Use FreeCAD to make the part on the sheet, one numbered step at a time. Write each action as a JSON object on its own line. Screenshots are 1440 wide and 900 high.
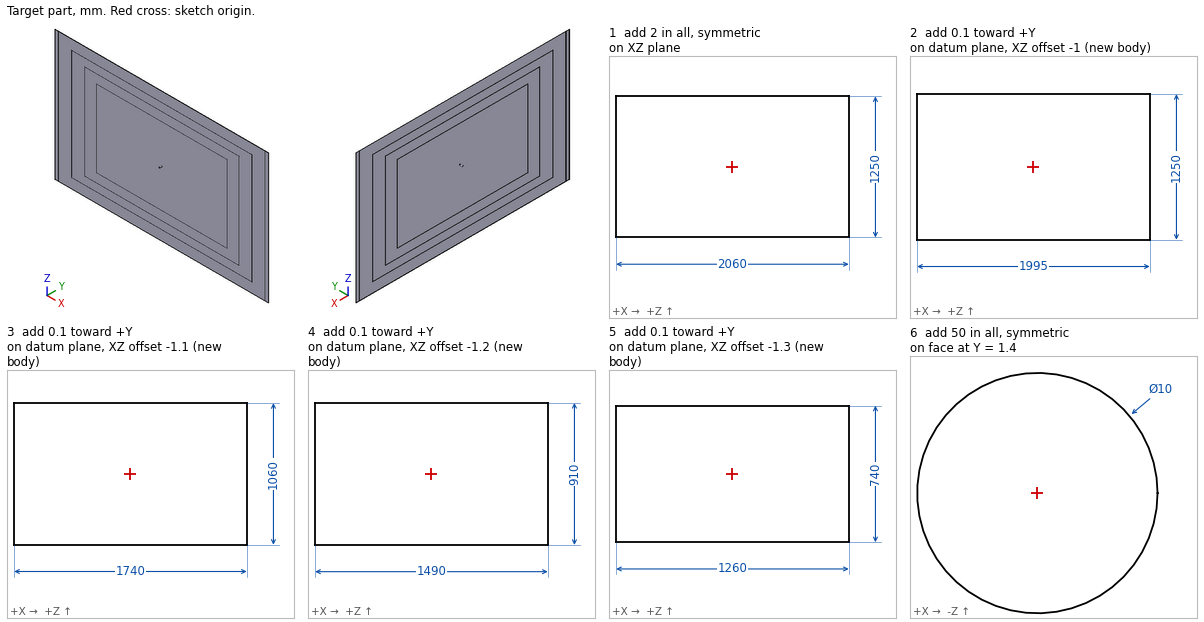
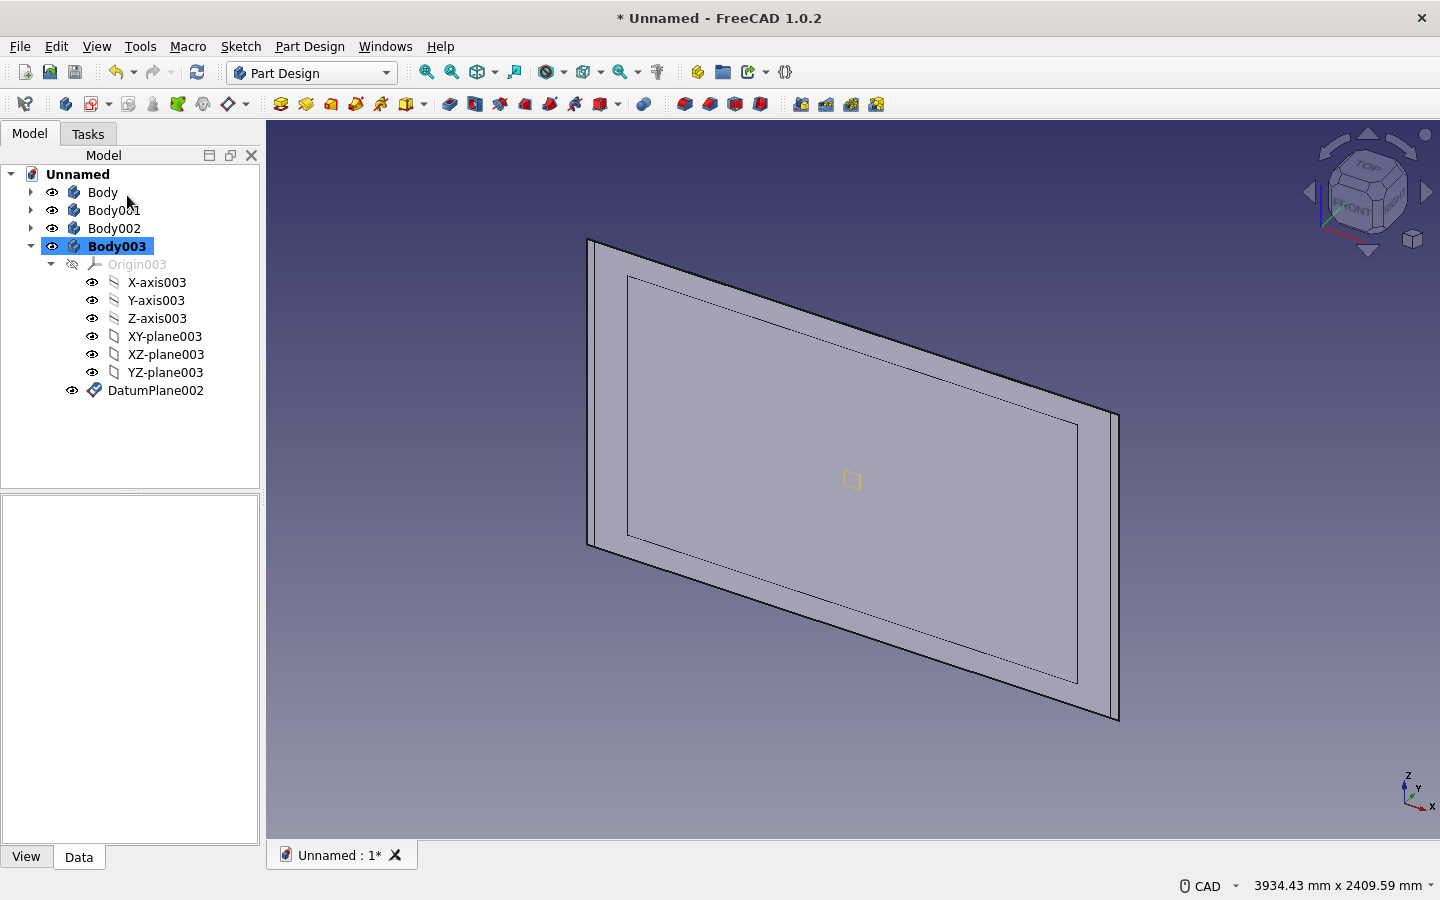
{"action": "left_click", "coordinate": [117, 390]}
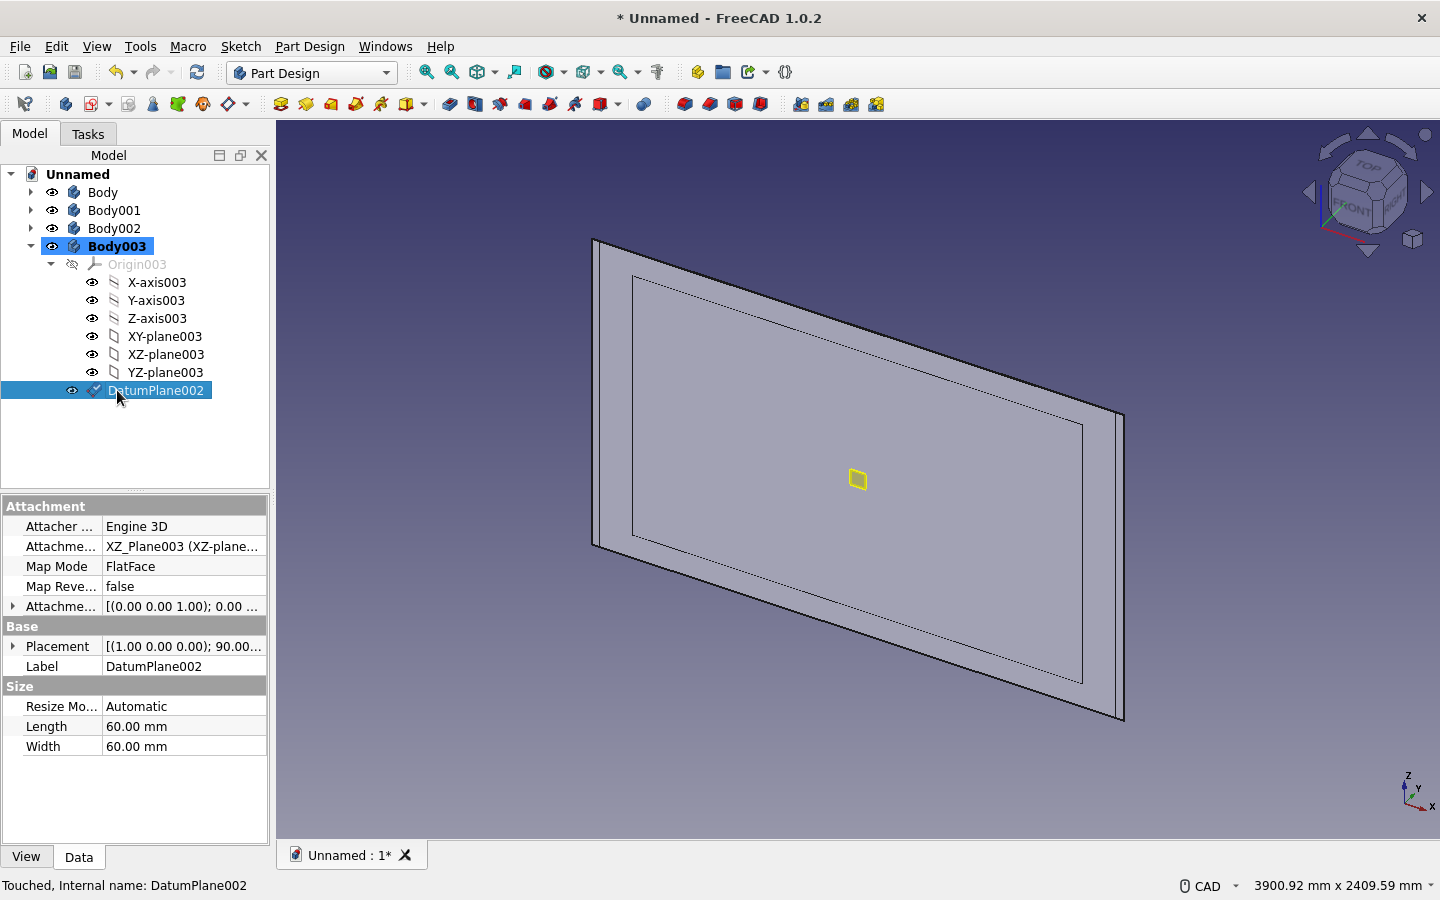
{"action": "left_click", "coordinate": [90, 104]}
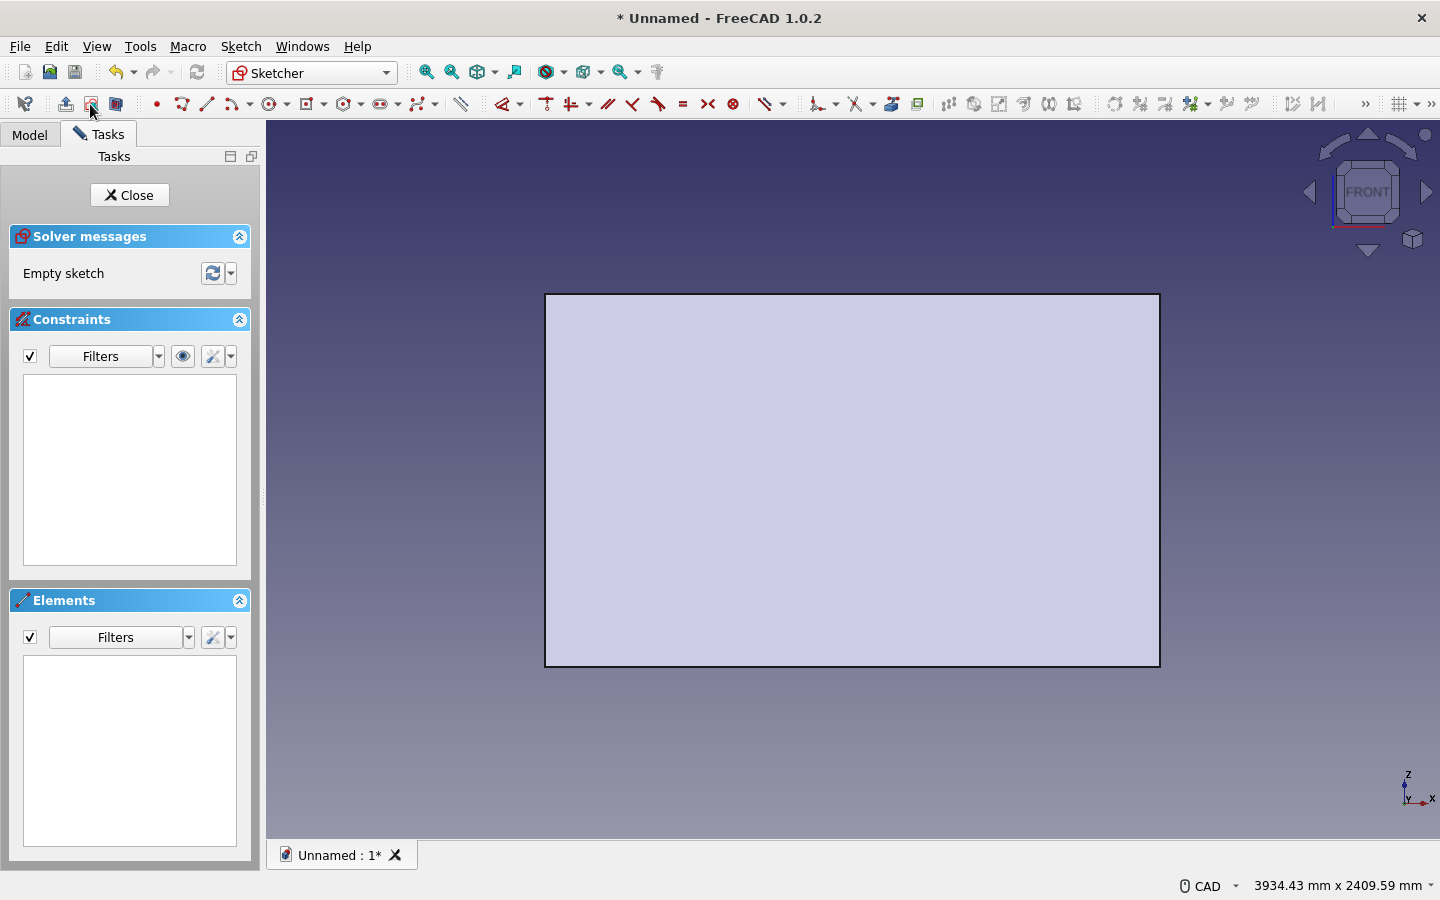
{"action": "scroll", "coordinate": [991, 481], "scroll_direction": "up", "scroll_amount": 2}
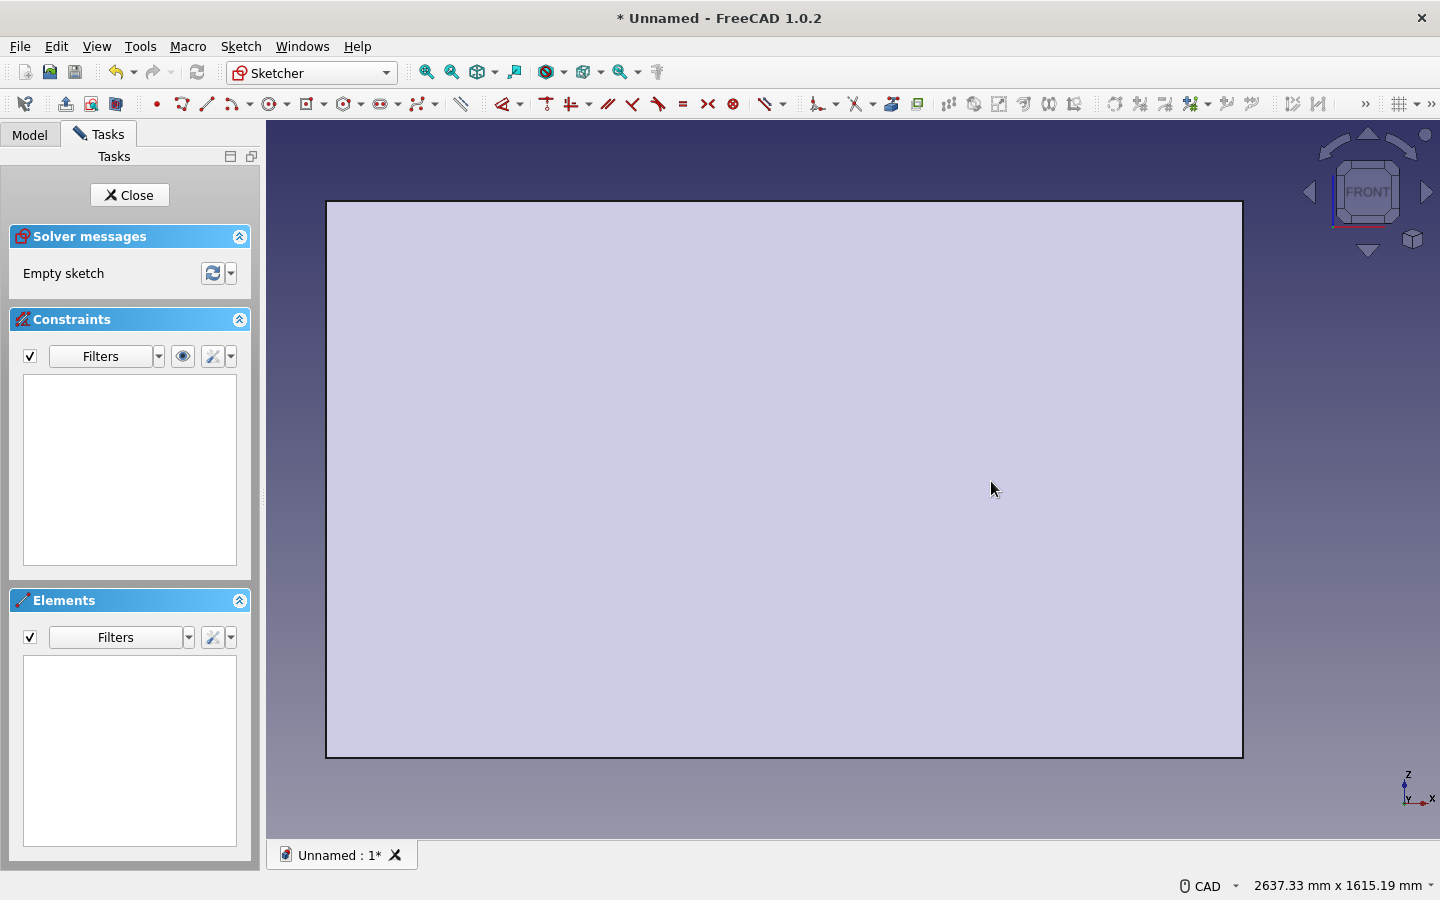
{"action": "left_click", "coordinate": [306, 104]}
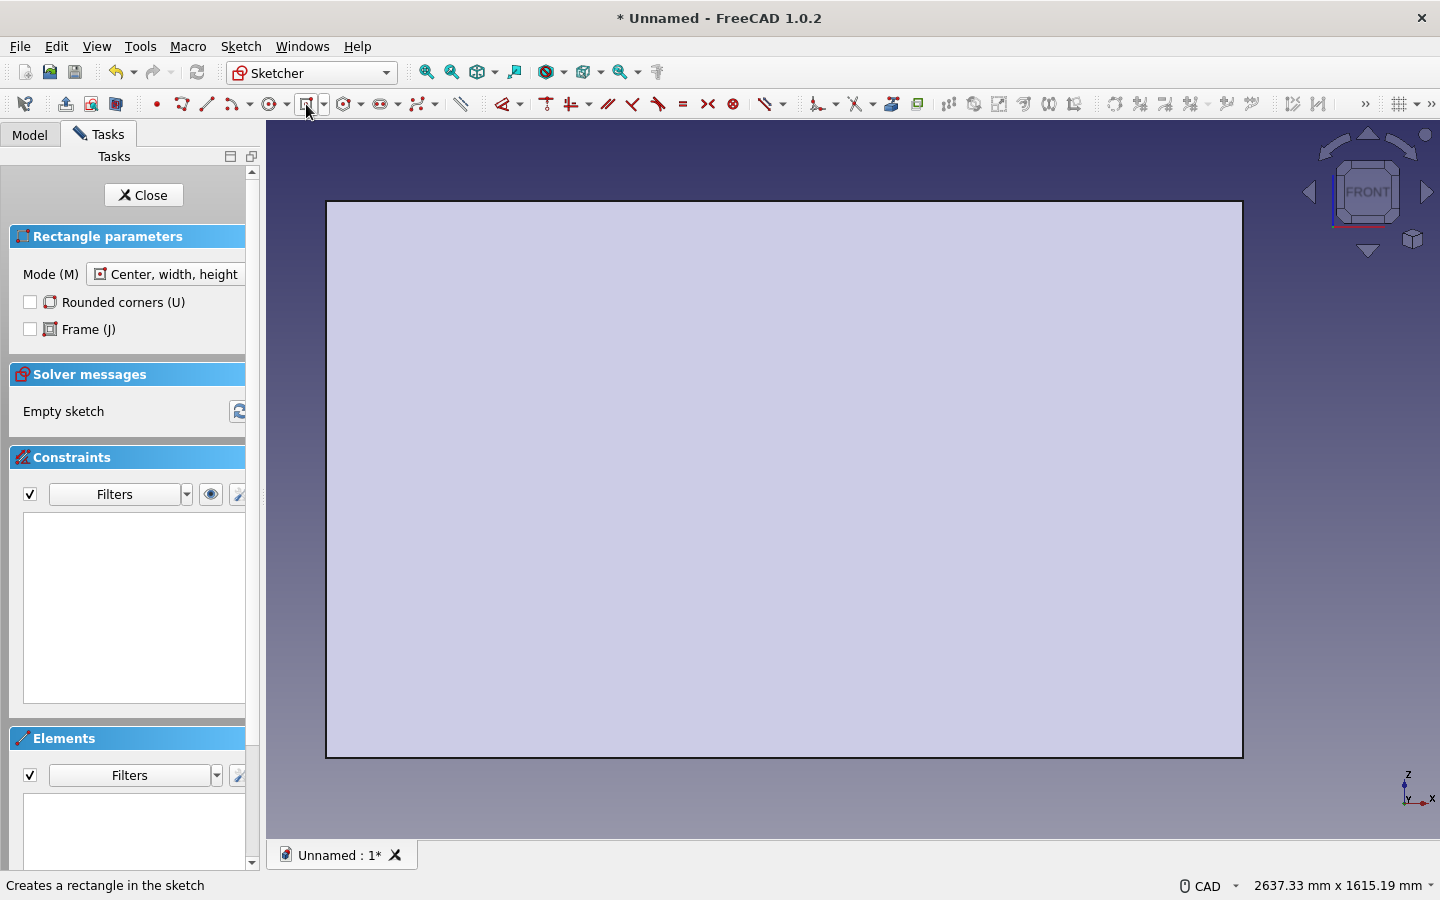
{"action": "left_click", "coordinate": [784, 479]}
{"action": "mouse_move", "coordinate": [1116, 277]}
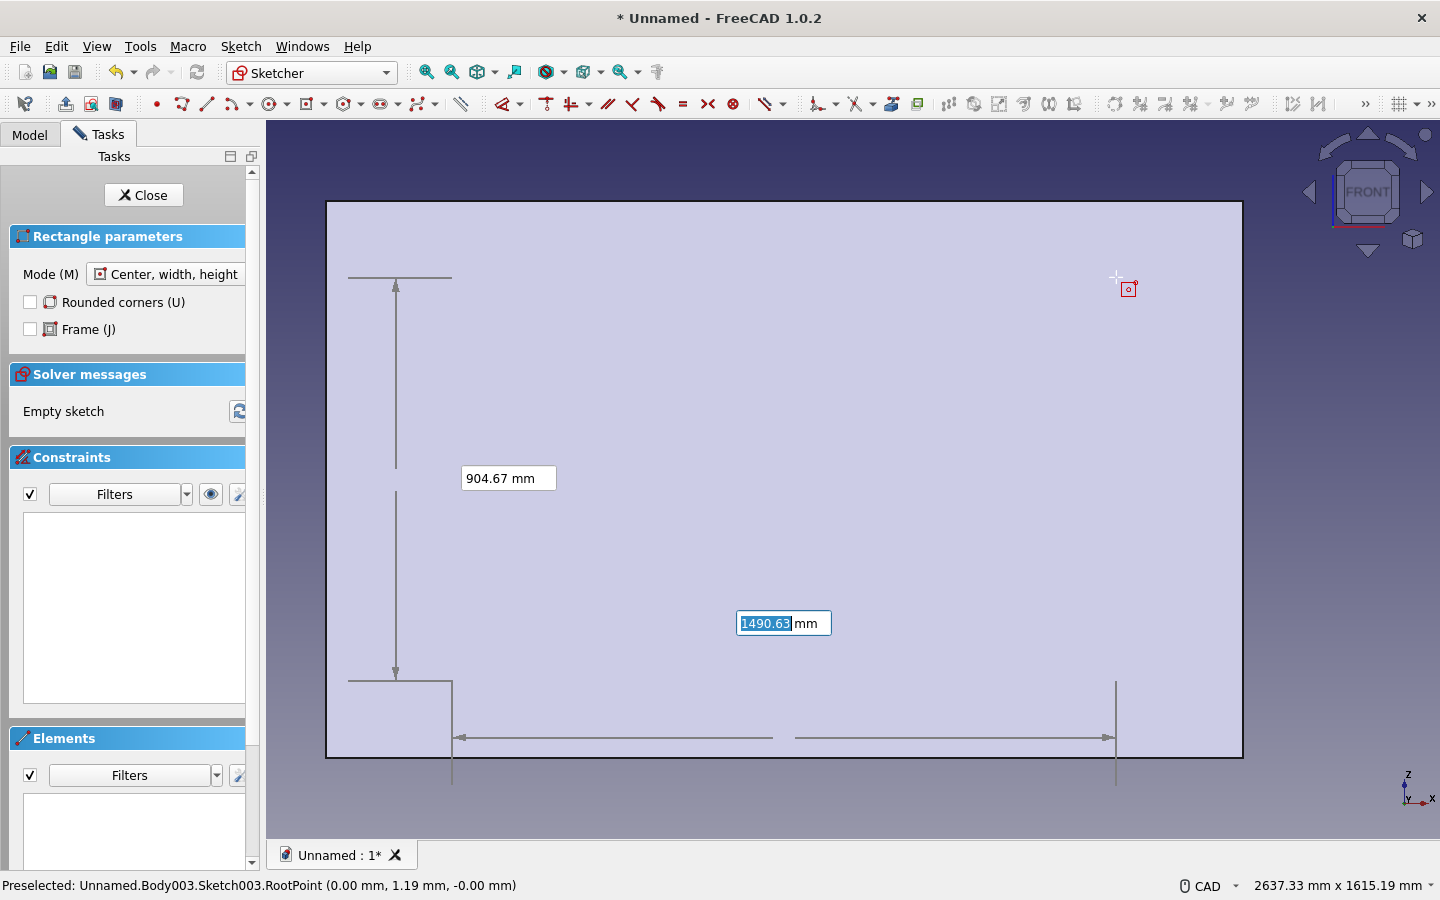
{"action": "type", "text": "1490"}
{"action": "key", "text": "Tab"}
{"action": "type", "text": "910"}
{"action": "key", "text": "Return"}
{"action": "key", "text": "Escape"}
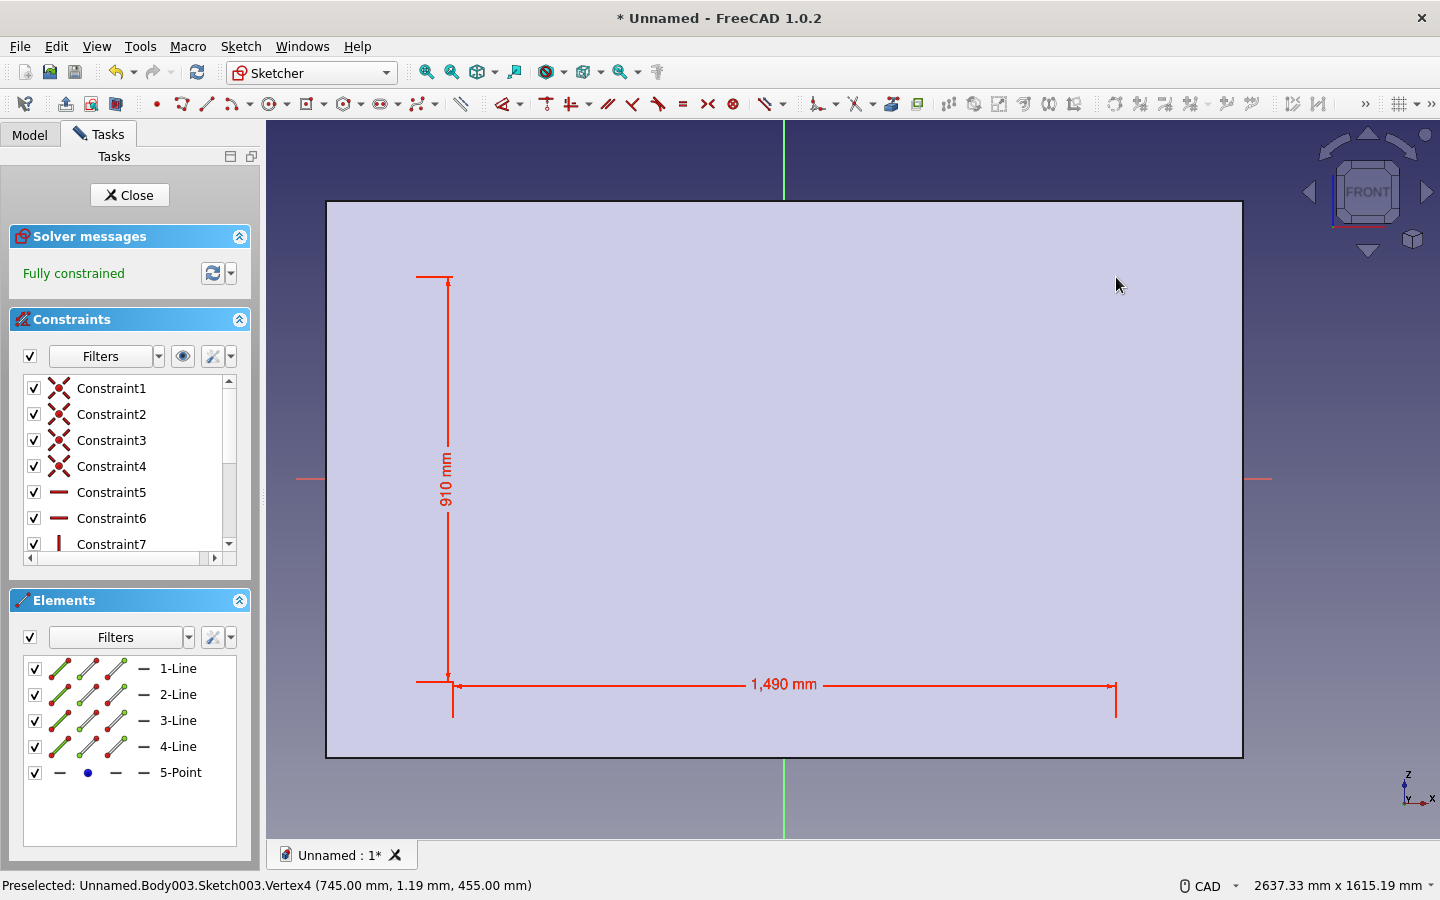
{"action": "left_click", "coordinate": [130, 195]}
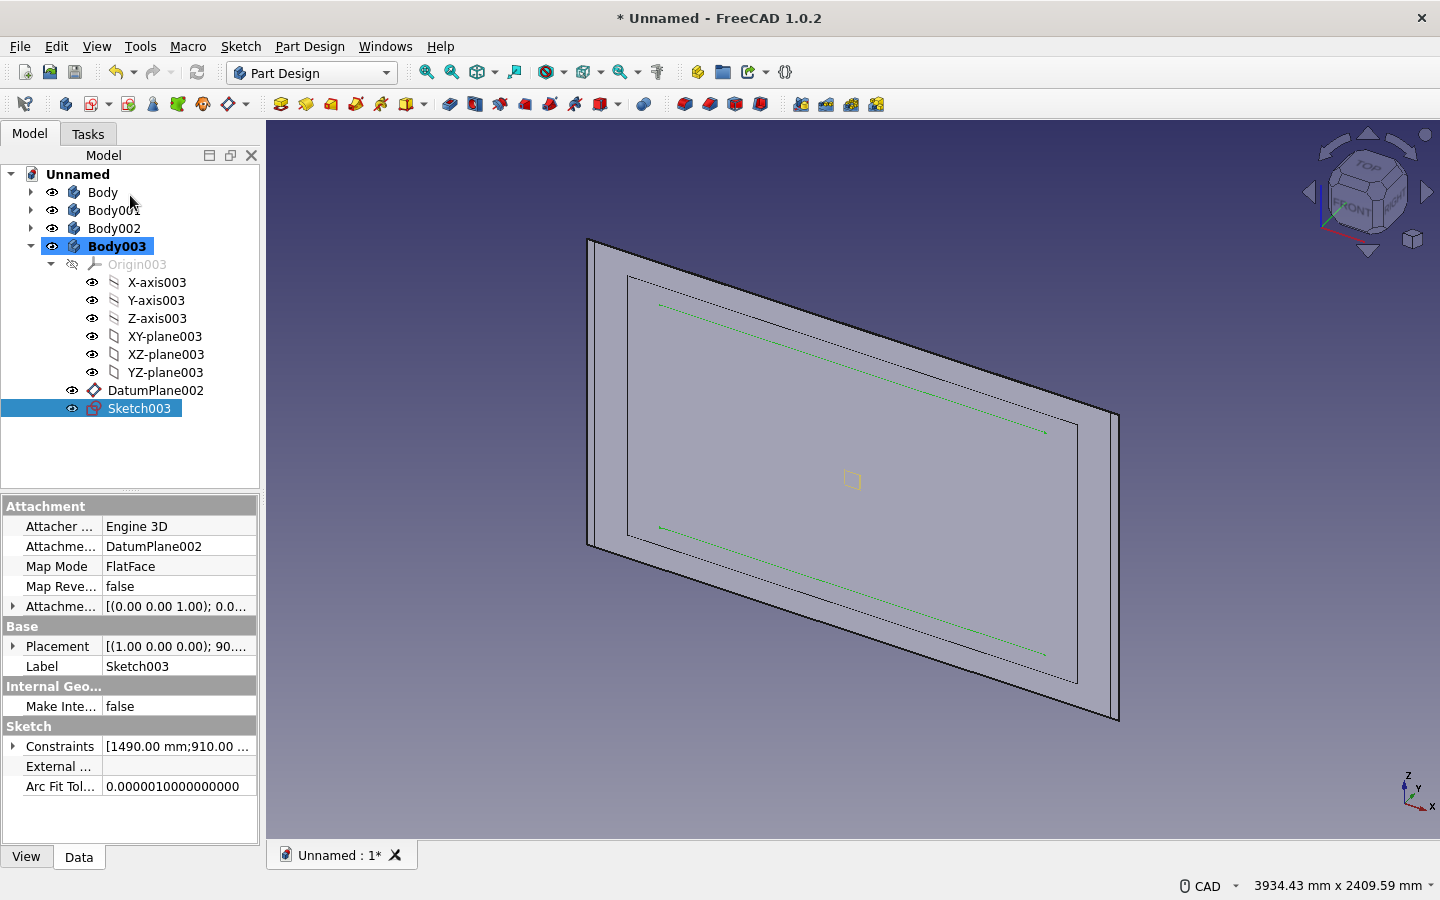
{"action": "left_click", "coordinate": [281, 104]}